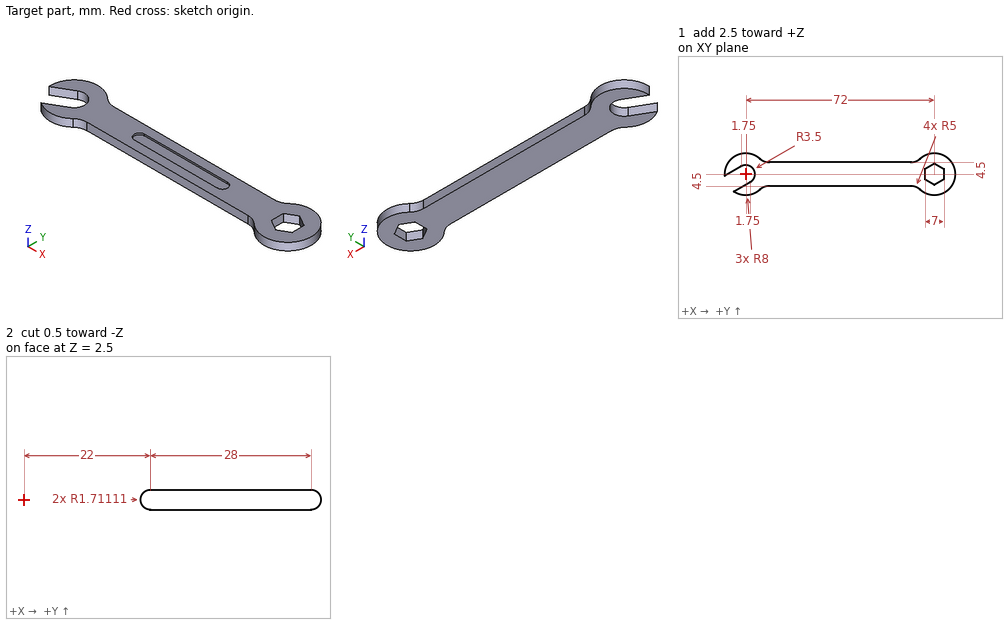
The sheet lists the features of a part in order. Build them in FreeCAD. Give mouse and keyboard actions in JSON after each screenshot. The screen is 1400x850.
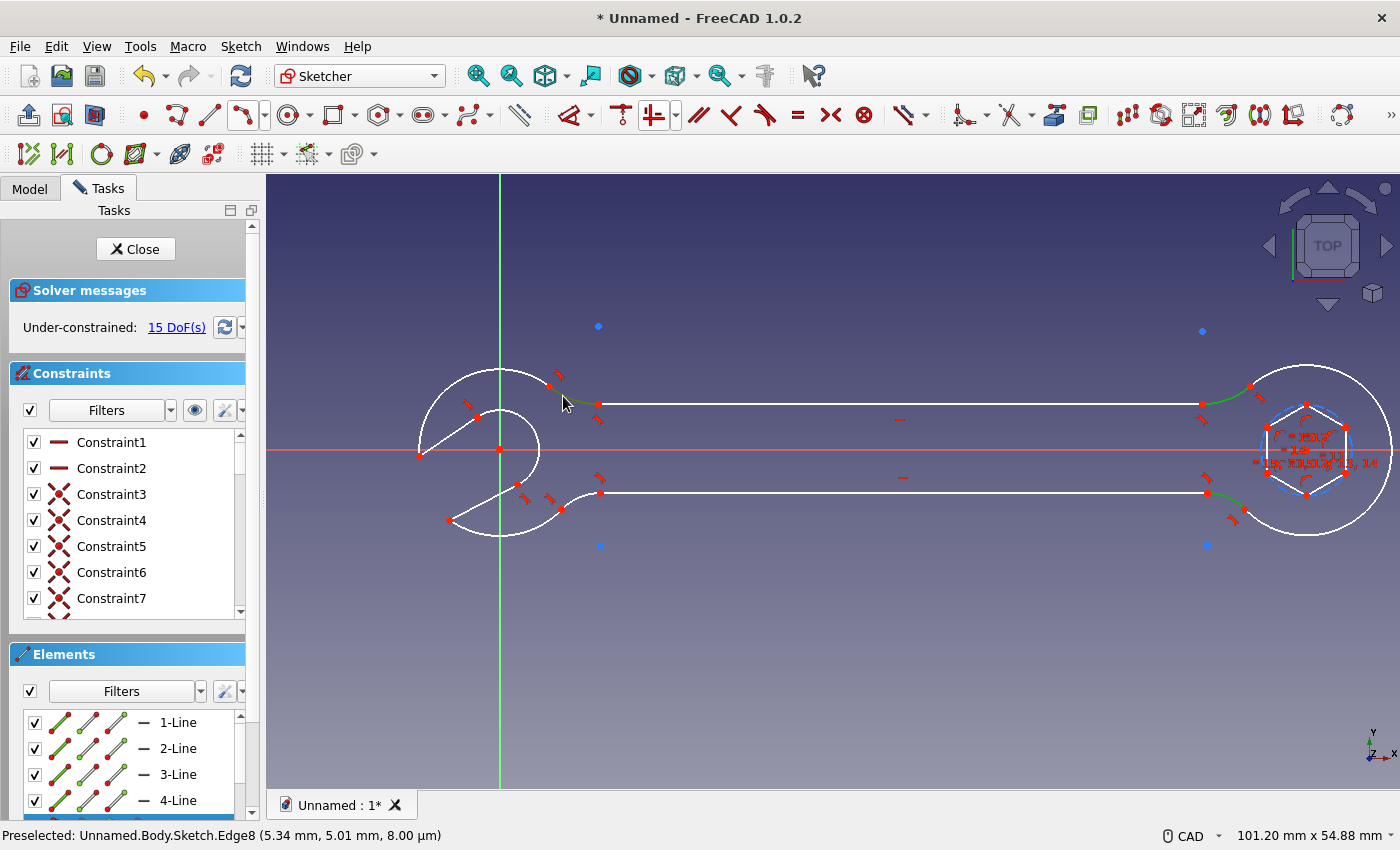
{"action": "left_click", "coordinate": [587, 495]}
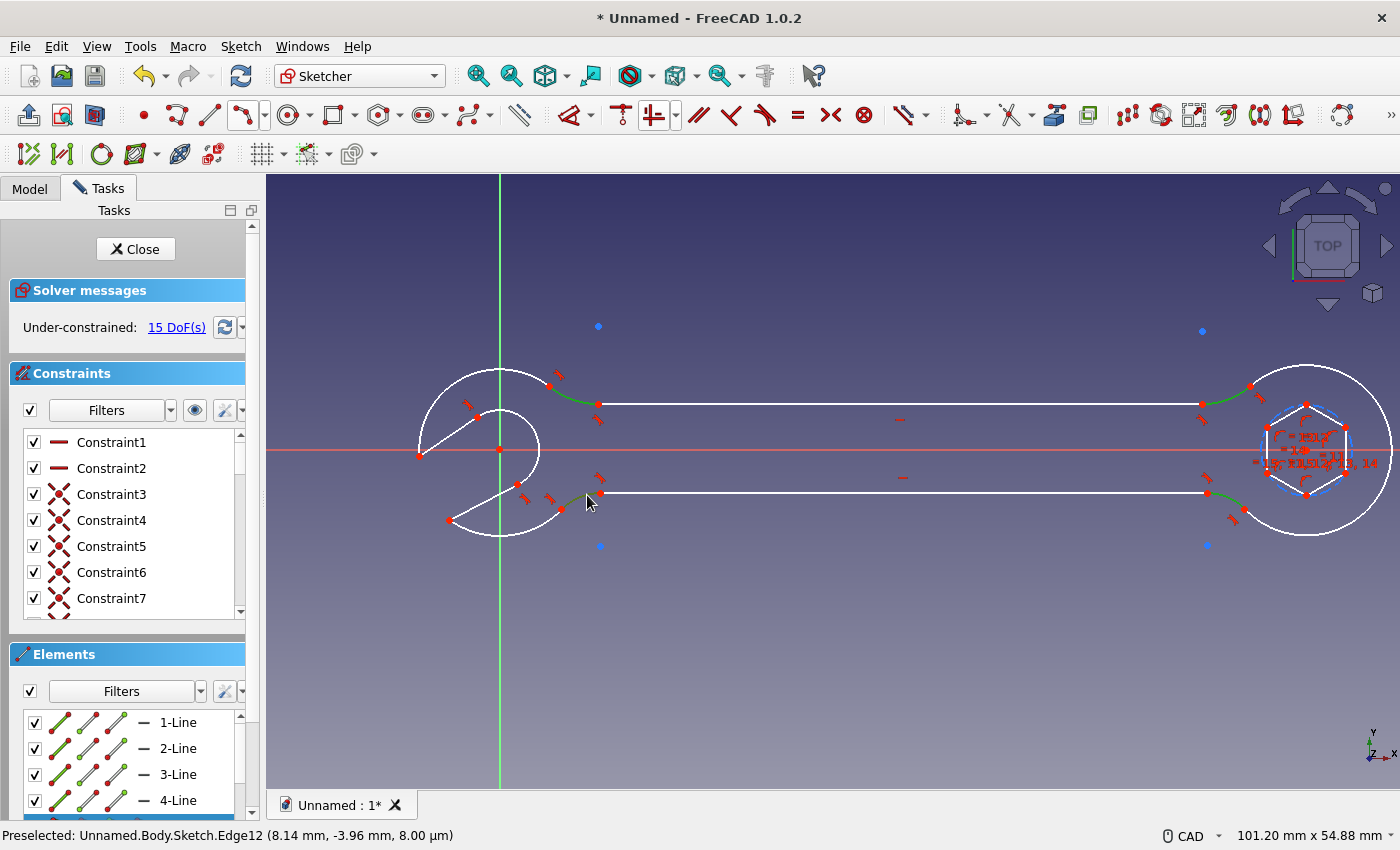
{"action": "key", "text": "e"}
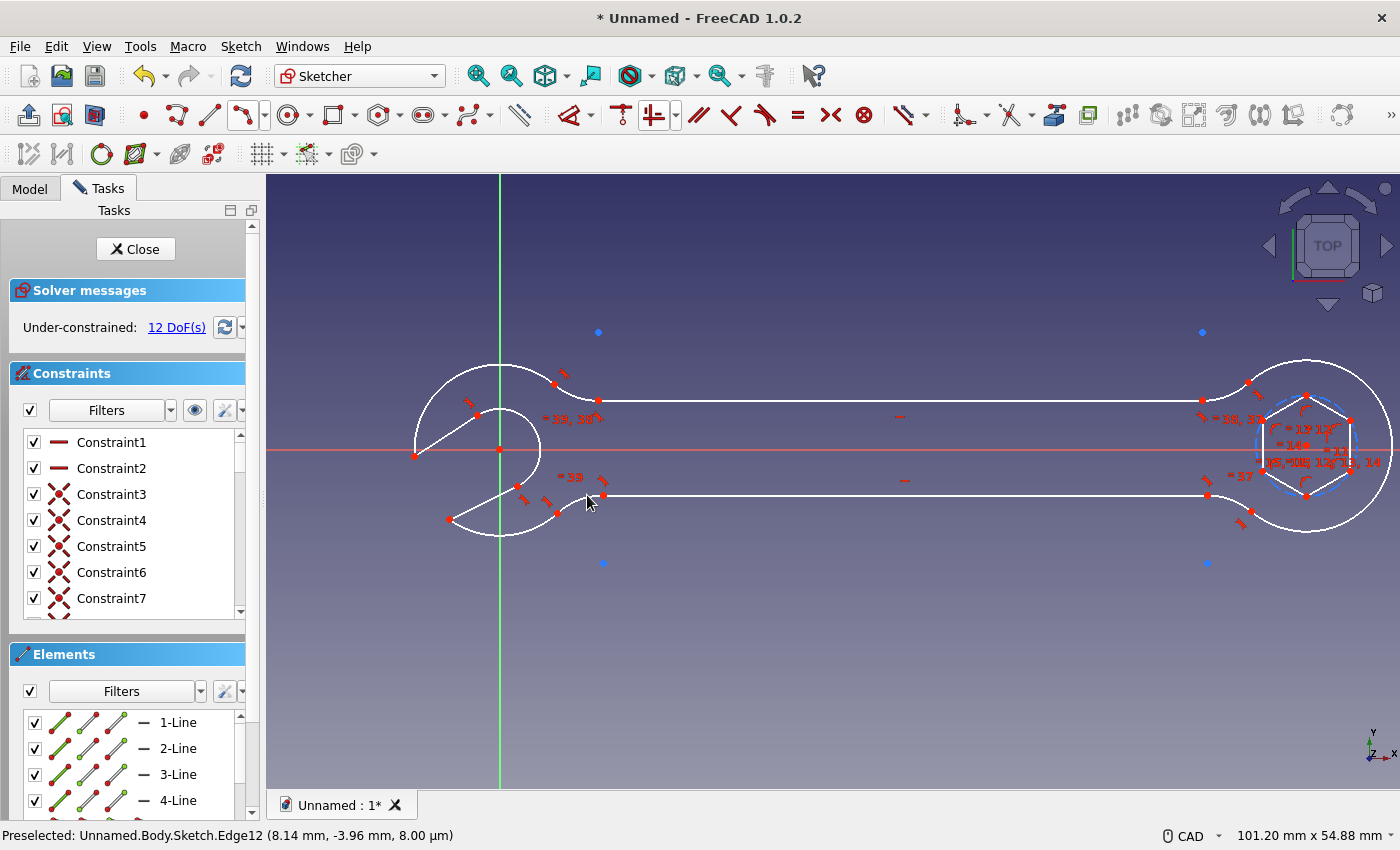
{"action": "scroll", "coordinate": [483, 538], "scroll_direction": "down", "scroll_amount": 2}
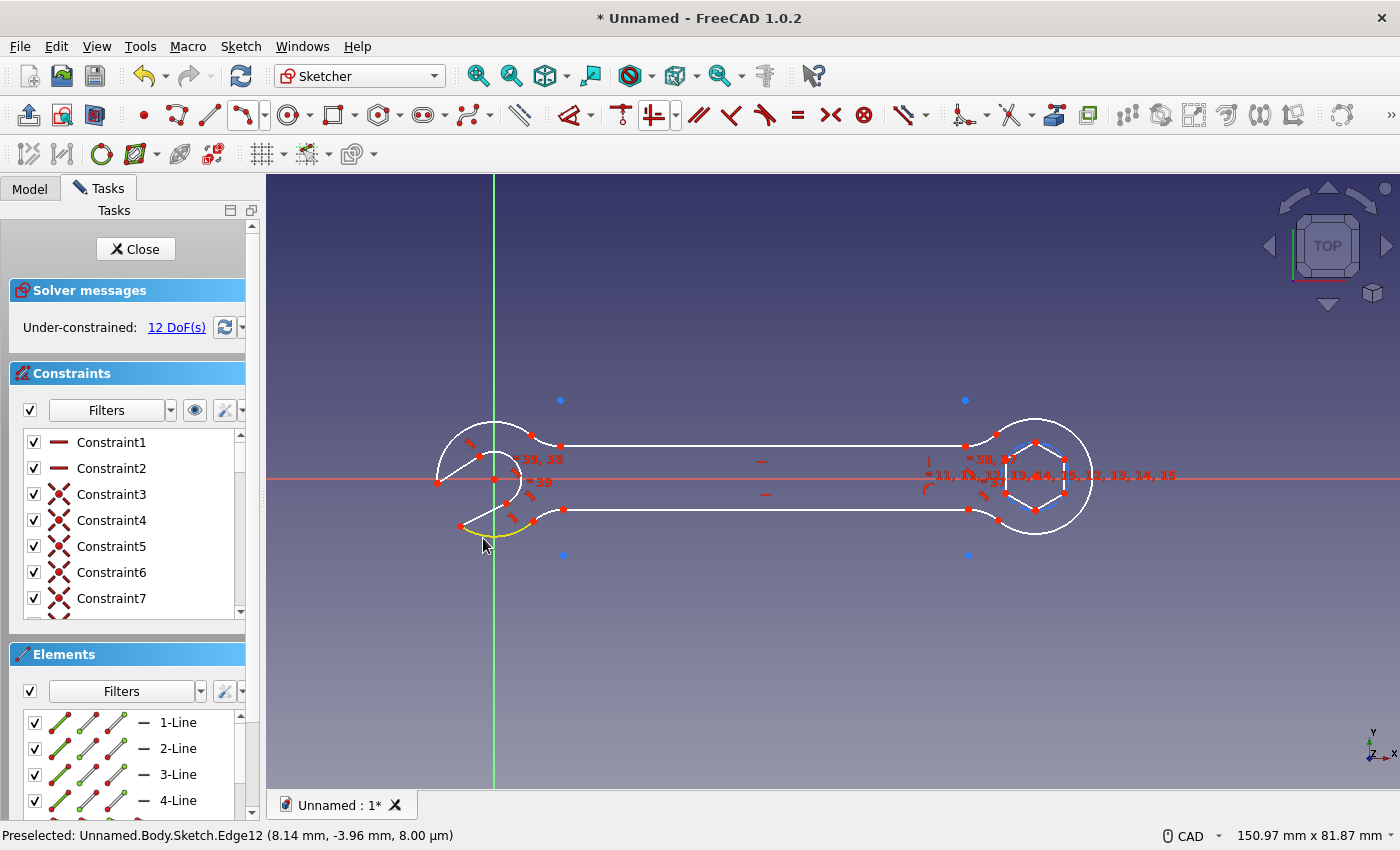
{"action": "left_click", "coordinate": [1071, 521]}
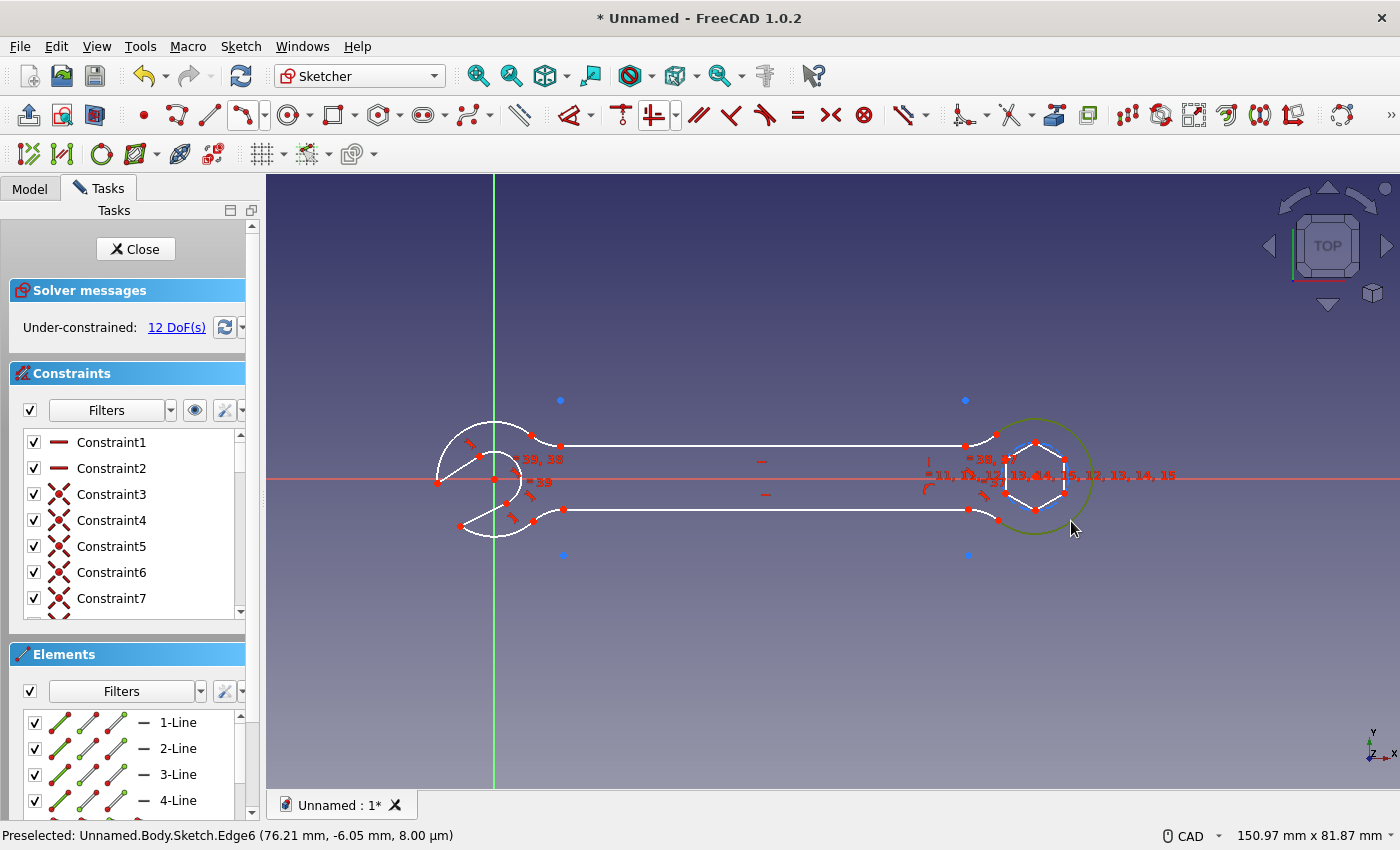
{"action": "left_click", "coordinate": [494, 422]}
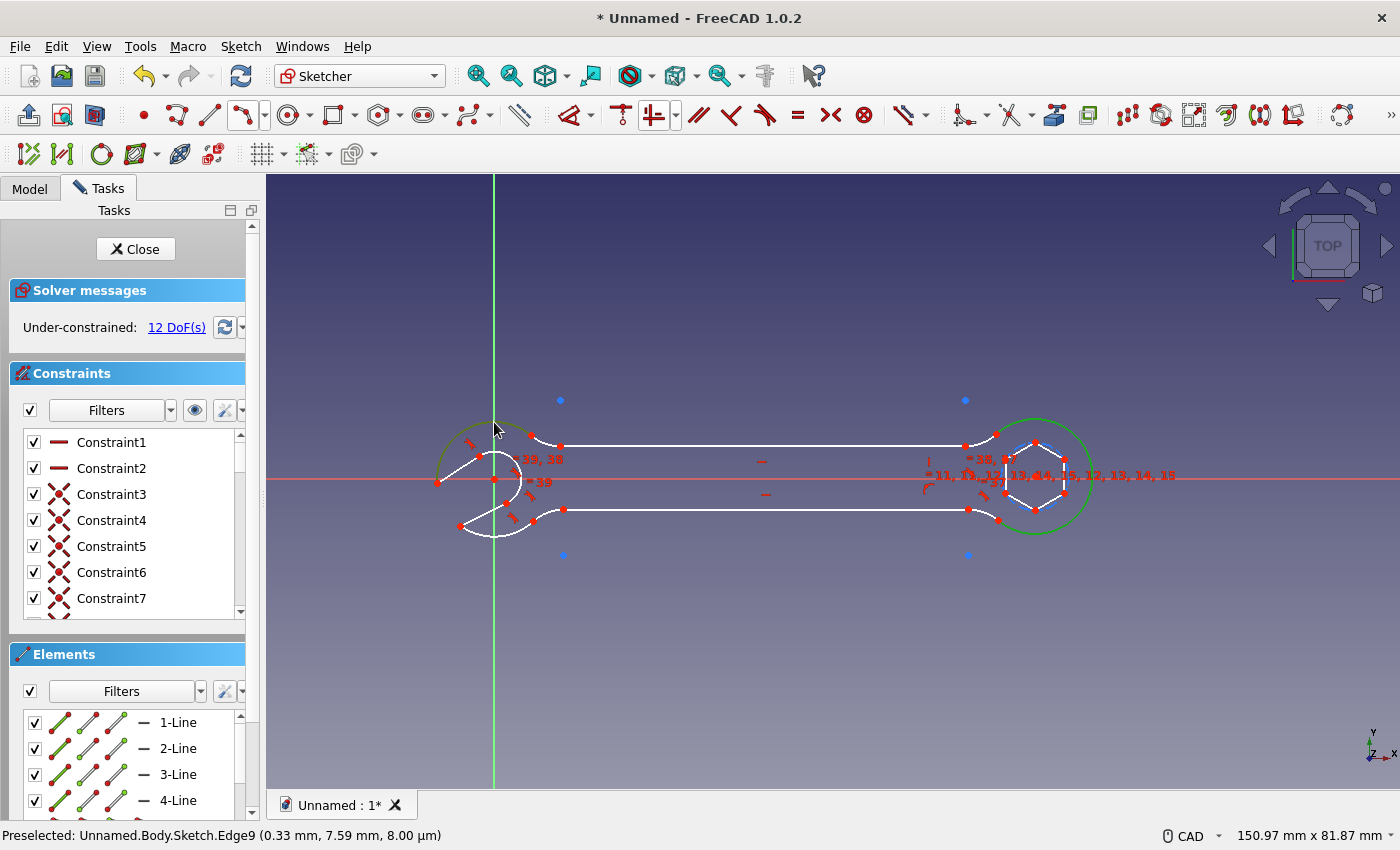
{"action": "left_click", "coordinate": [482, 535]}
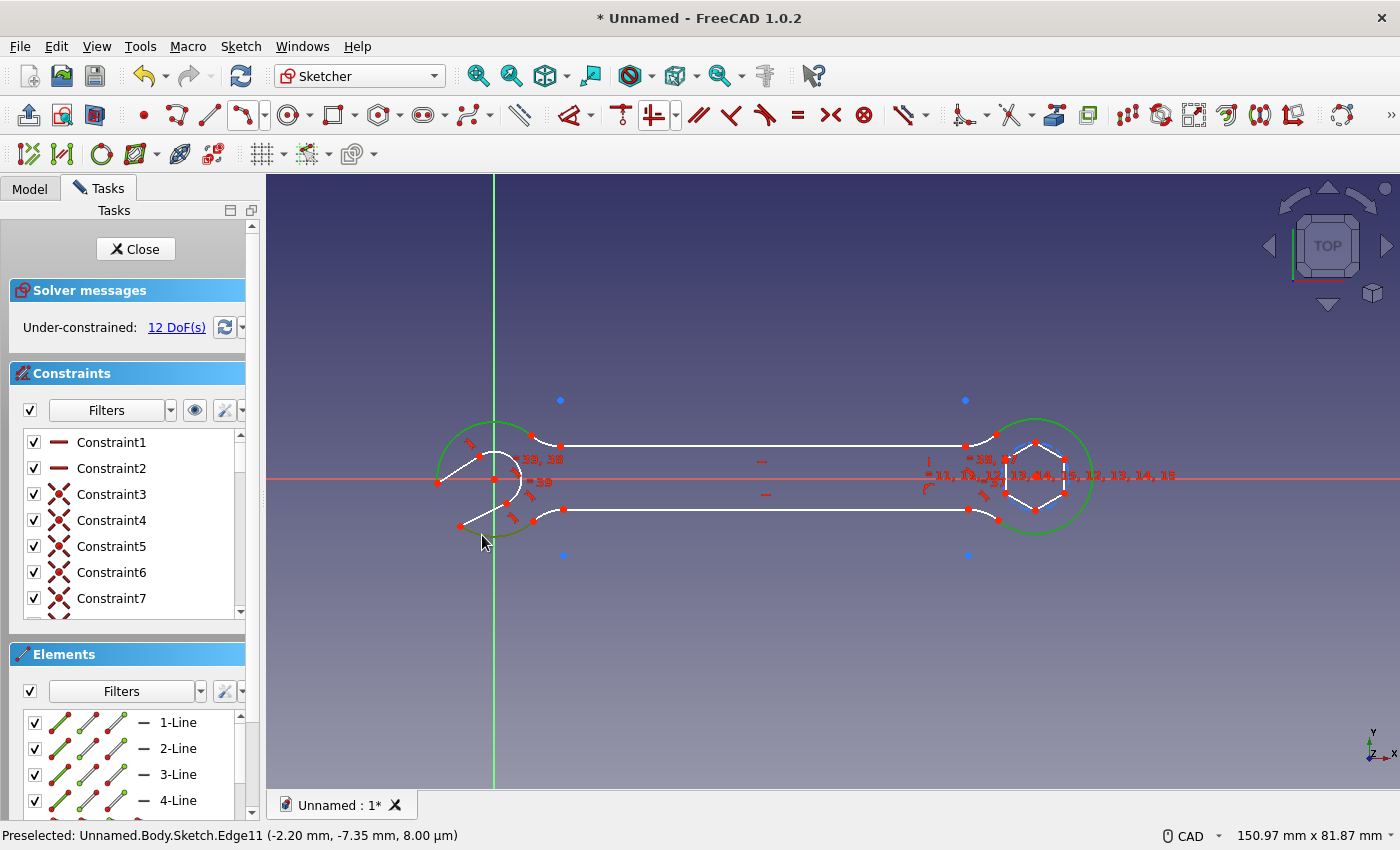
{"action": "left_click", "coordinate": [798, 116]}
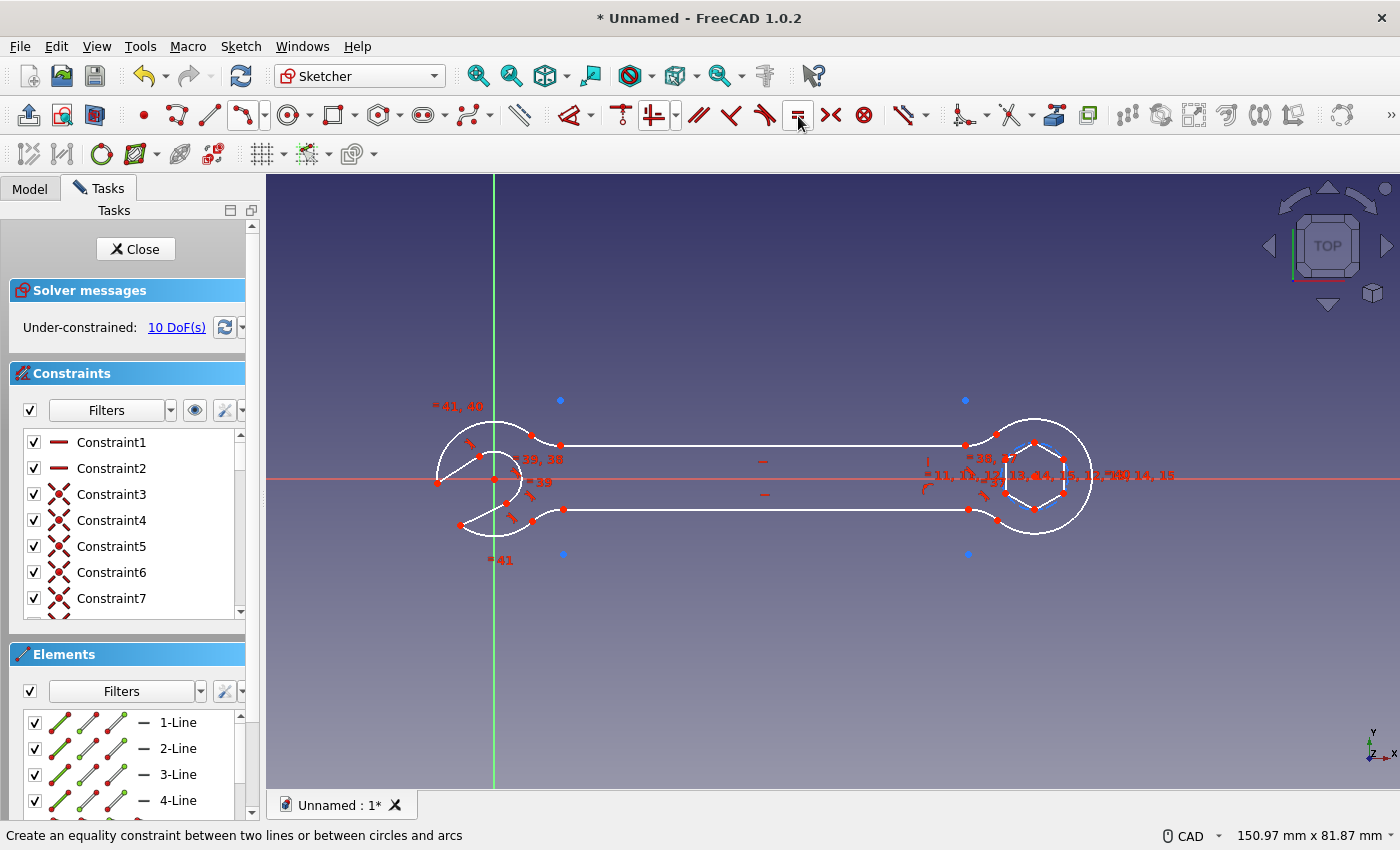
{"action": "left_click", "coordinate": [1035, 476]}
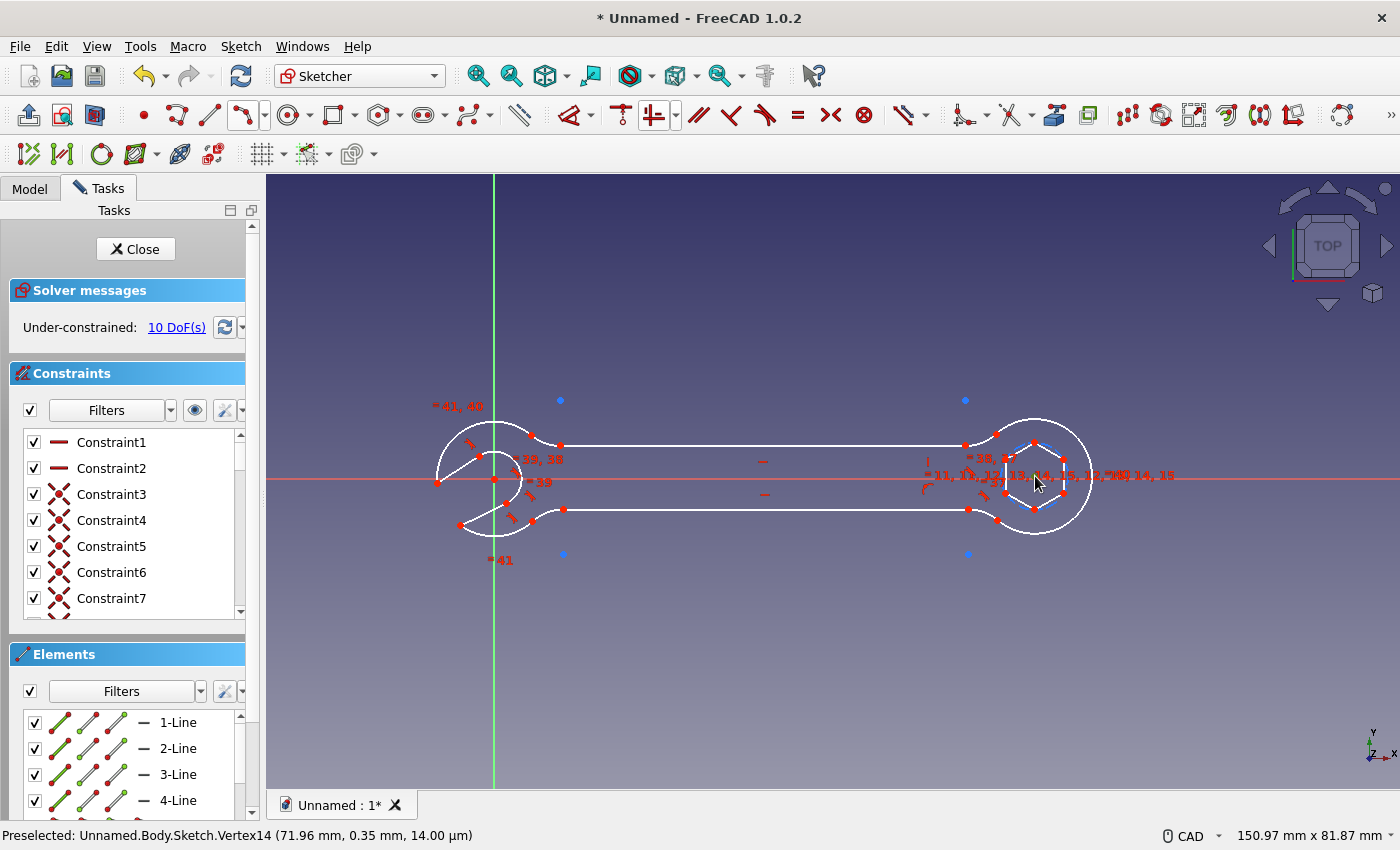
{"action": "left_click", "coordinate": [361, 479]}